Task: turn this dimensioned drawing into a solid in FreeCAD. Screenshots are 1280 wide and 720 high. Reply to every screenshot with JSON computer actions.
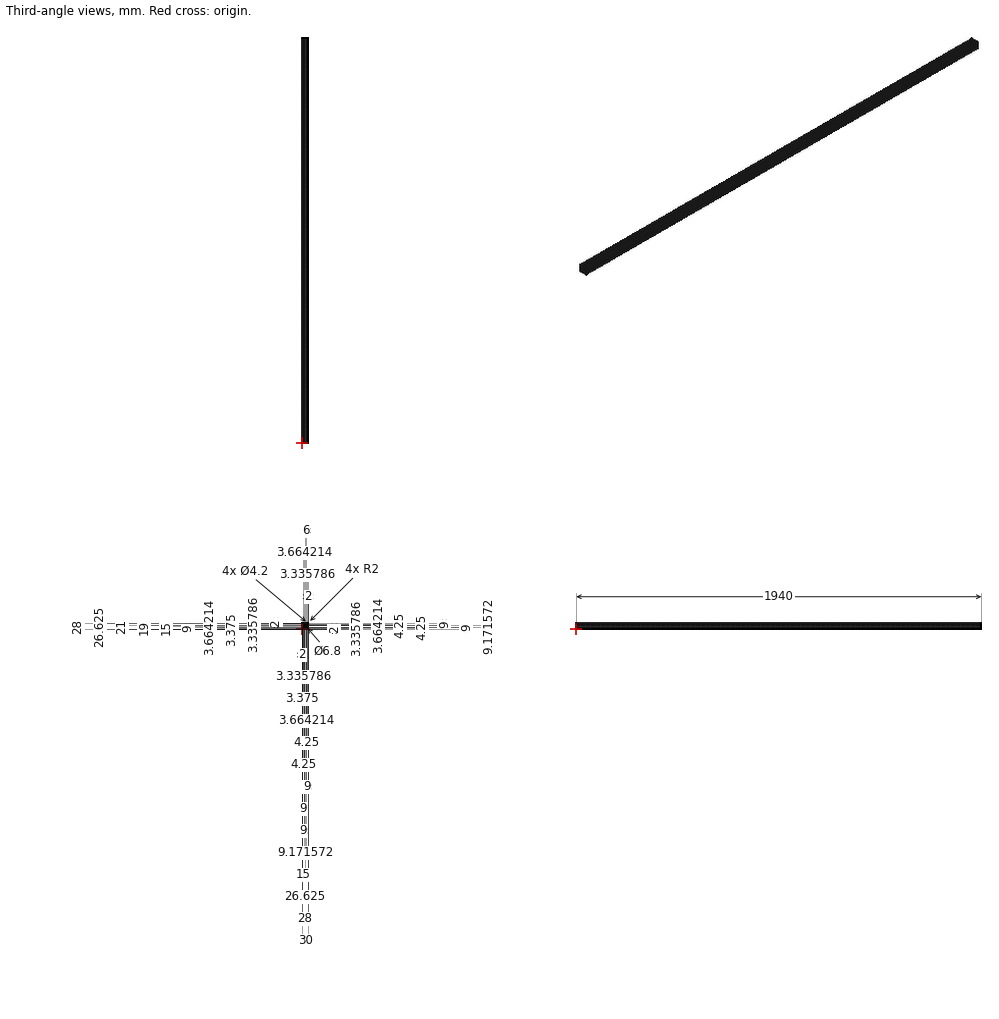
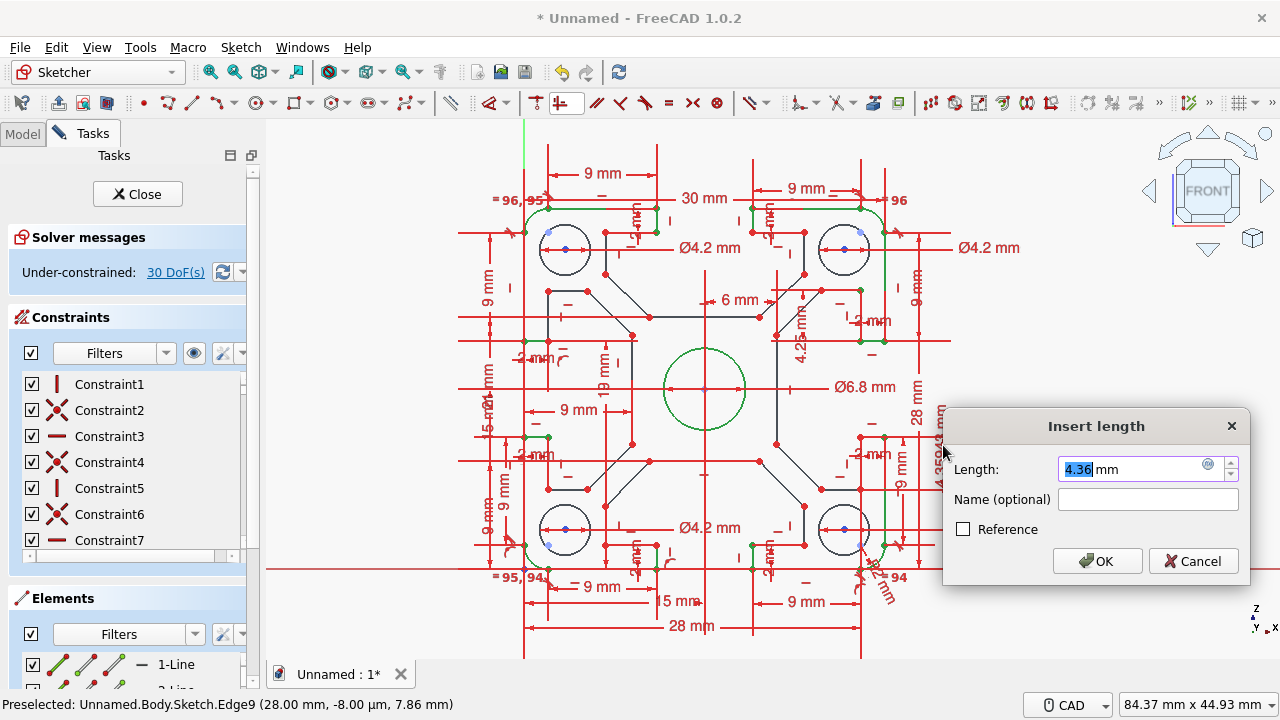
{"action": "type", "text": "4.25"}
{"action": "key", "text": "Return"}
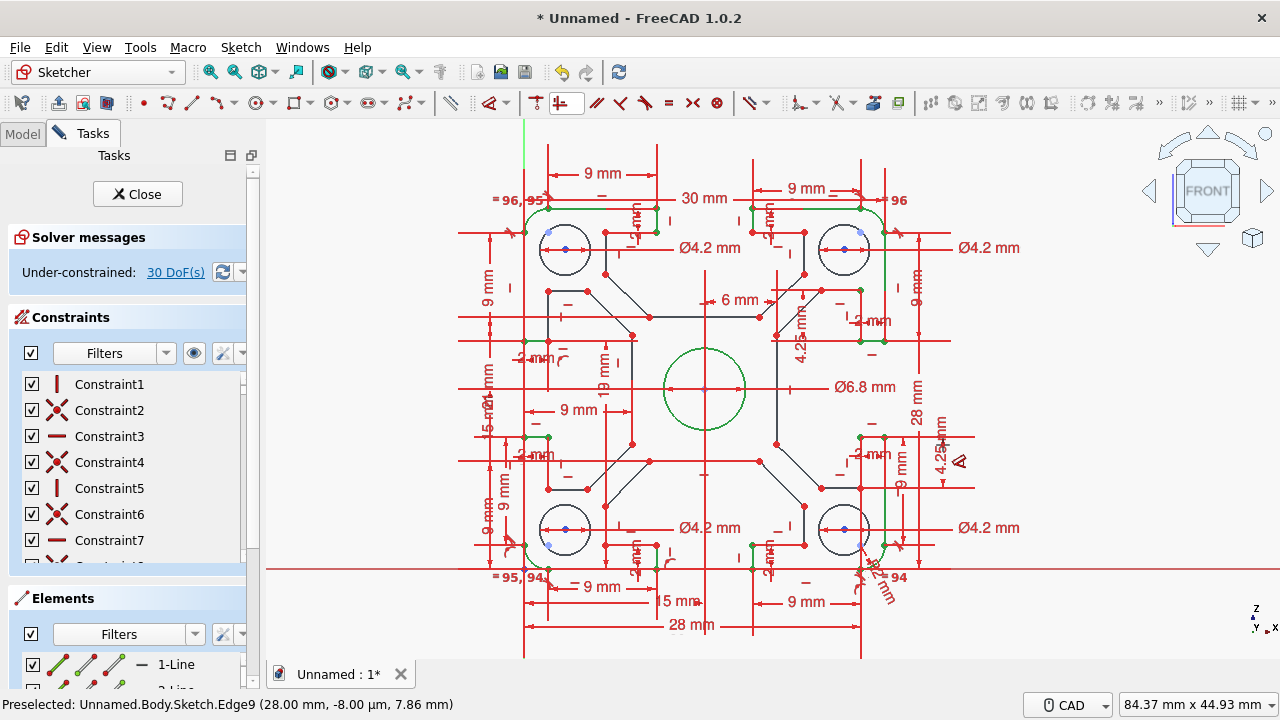
{"action": "left_click", "coordinate": [768, 545]}
{"action": "left_click", "coordinate": [778, 511]}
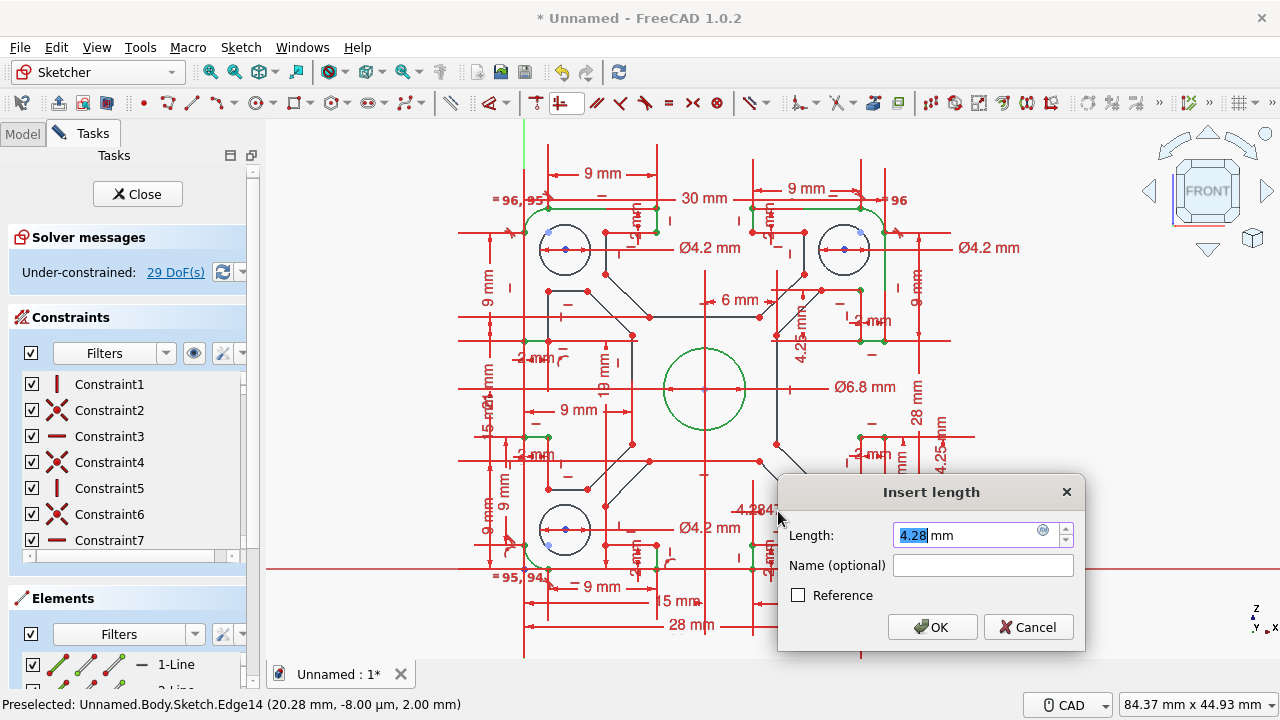
{"action": "type", "text": "4.25"}
{"action": "key", "text": "Return"}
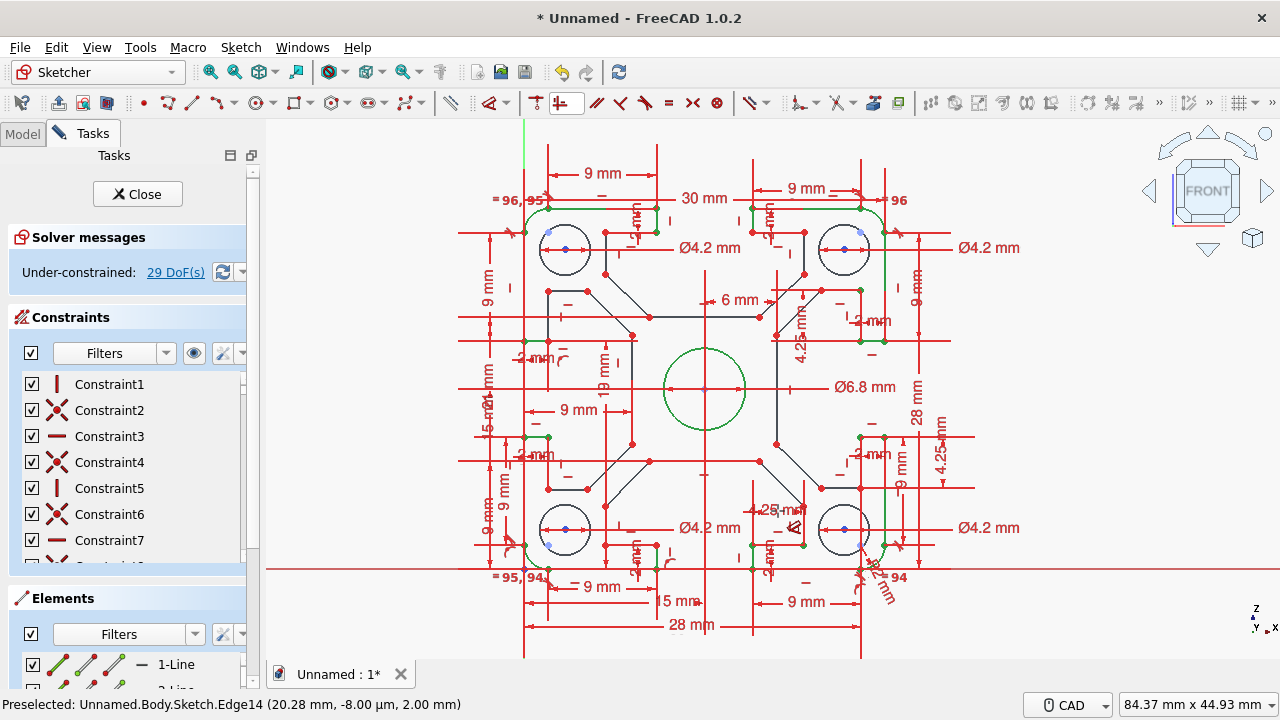
{"action": "left_click", "coordinate": [621, 545]}
{"action": "left_click", "coordinate": [631, 511]}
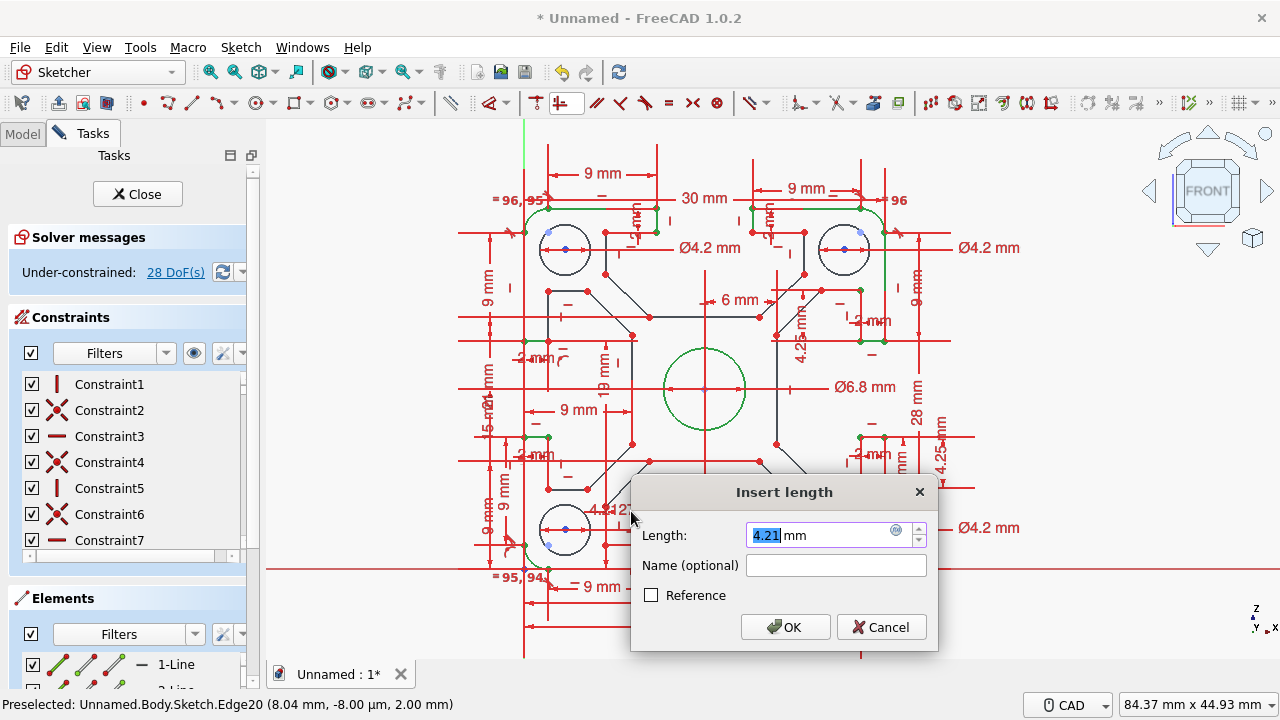
{"action": "type", "text": "4.25"}
{"action": "key", "text": "Return"}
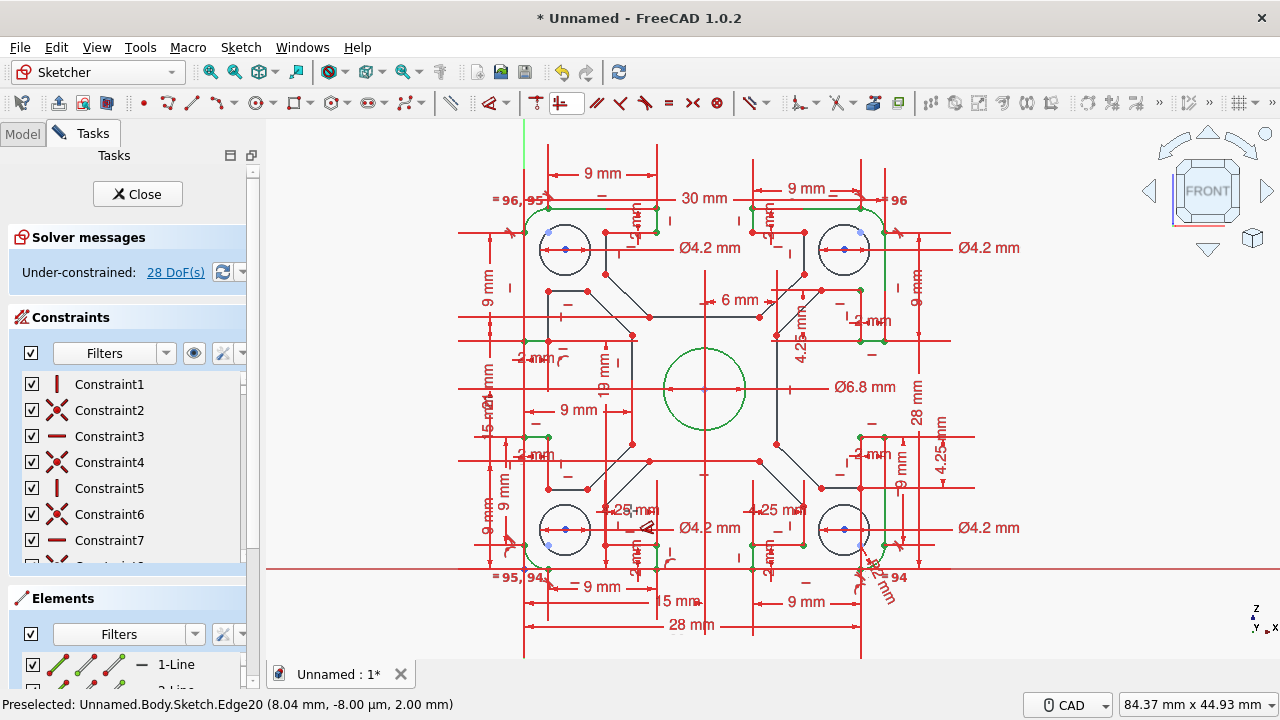
{"action": "left_click", "coordinate": [548, 453]}
{"action": "left_click", "coordinate": [606, 451]}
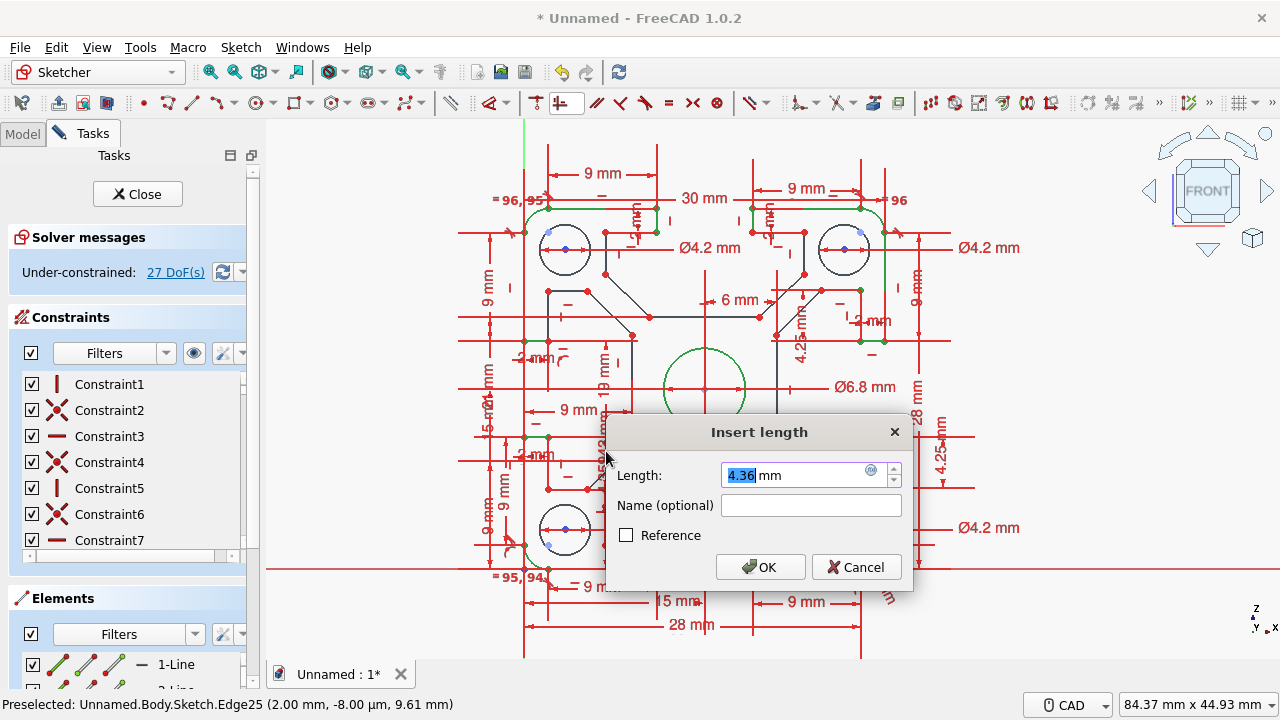
{"action": "type", "text": "4.25"}
{"action": "key", "text": "Return"}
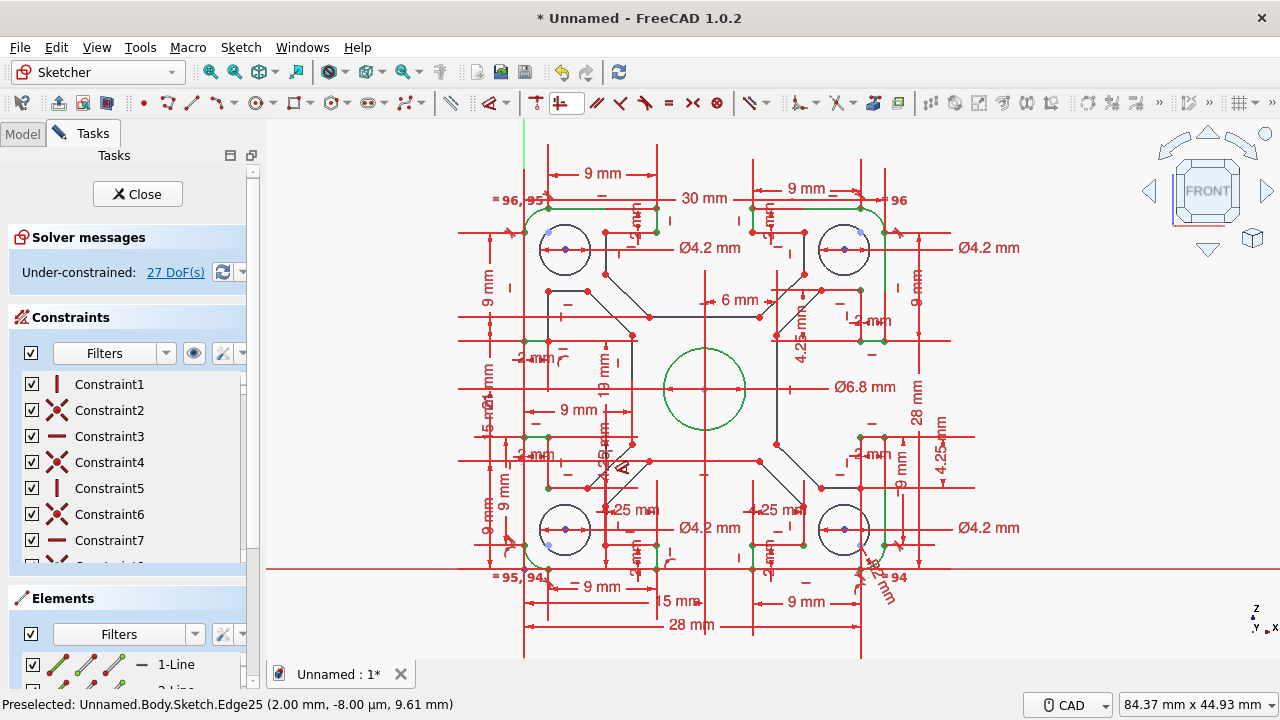
{"action": "left_click", "coordinate": [548, 306]}
{"action": "left_click", "coordinate": [582, 316]}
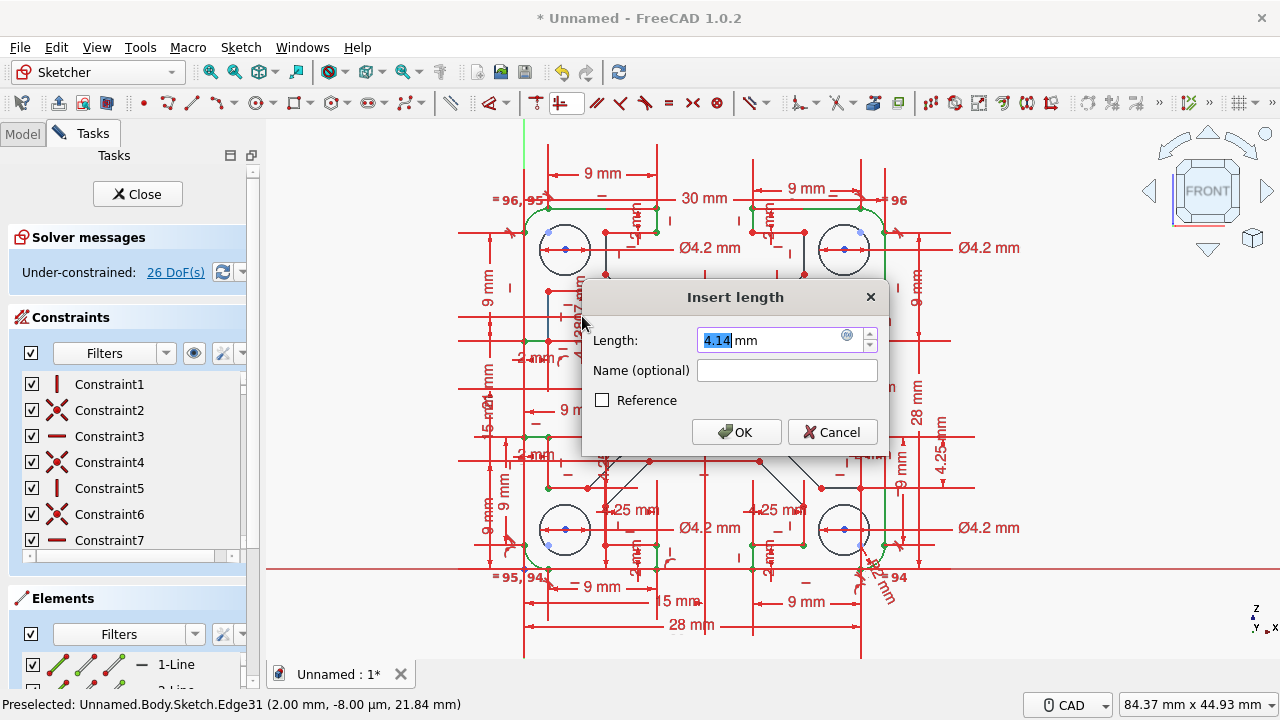
{"action": "type", "text": "4.25"}
{"action": "key", "text": "Return"}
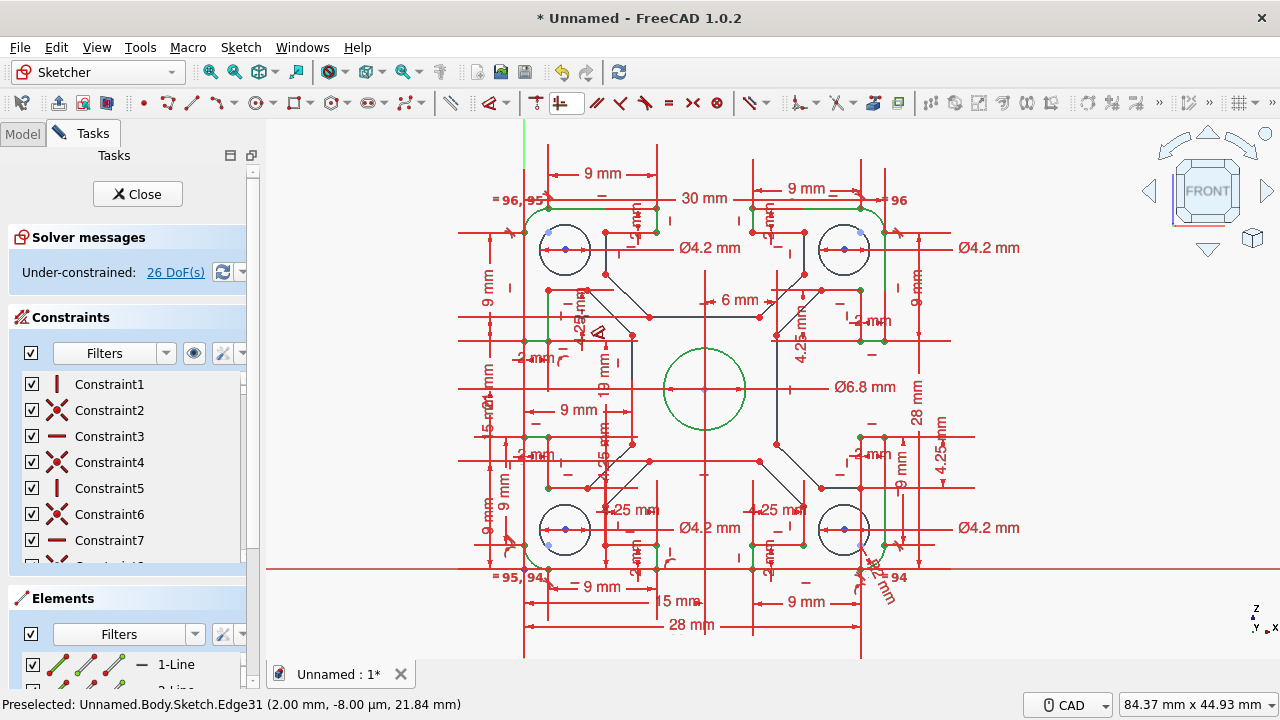
{"action": "left_click", "coordinate": [641, 233]}
{"action": "left_click", "coordinate": [631, 267]}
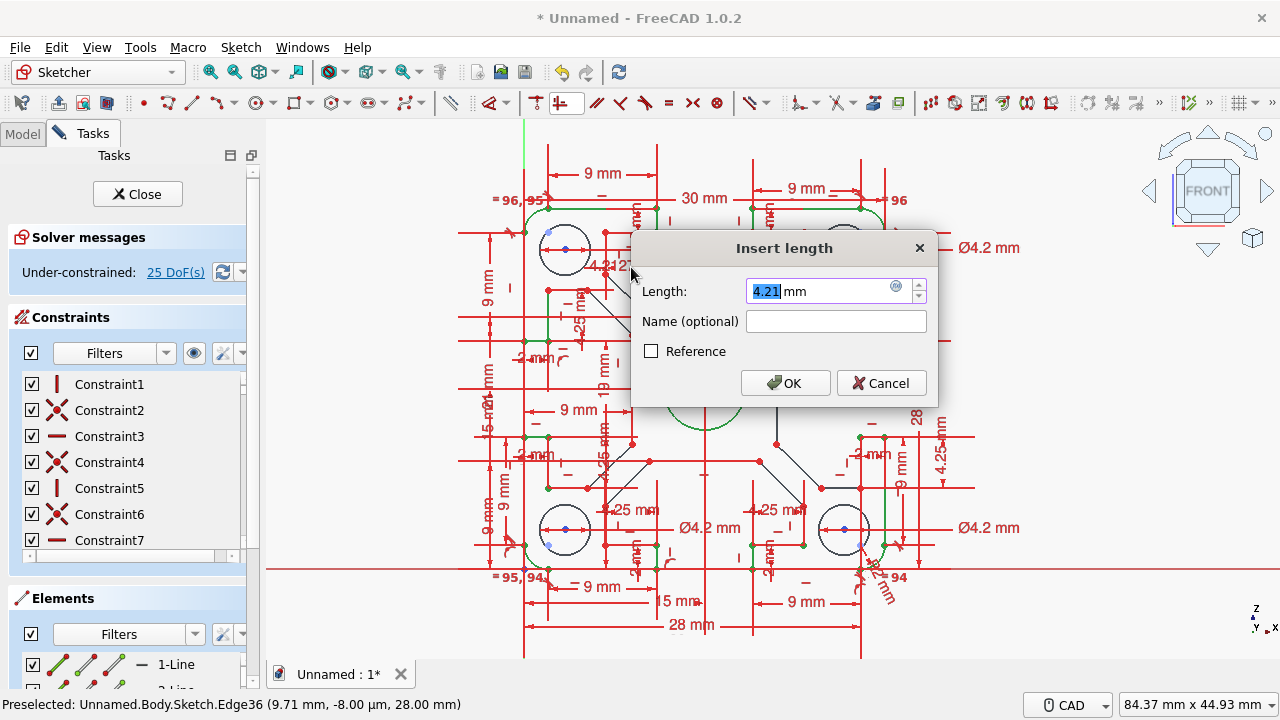
{"action": "type", "text": "4.25"}
{"action": "key", "text": "Return"}